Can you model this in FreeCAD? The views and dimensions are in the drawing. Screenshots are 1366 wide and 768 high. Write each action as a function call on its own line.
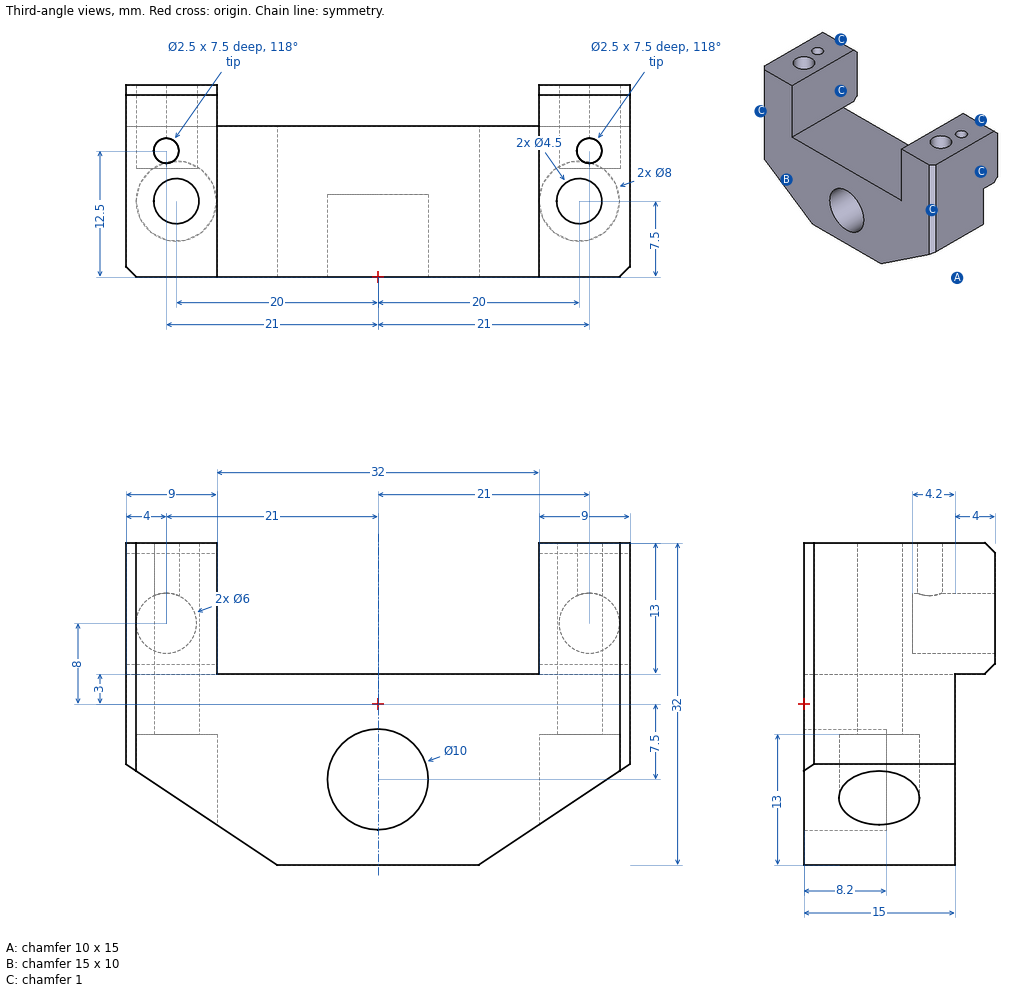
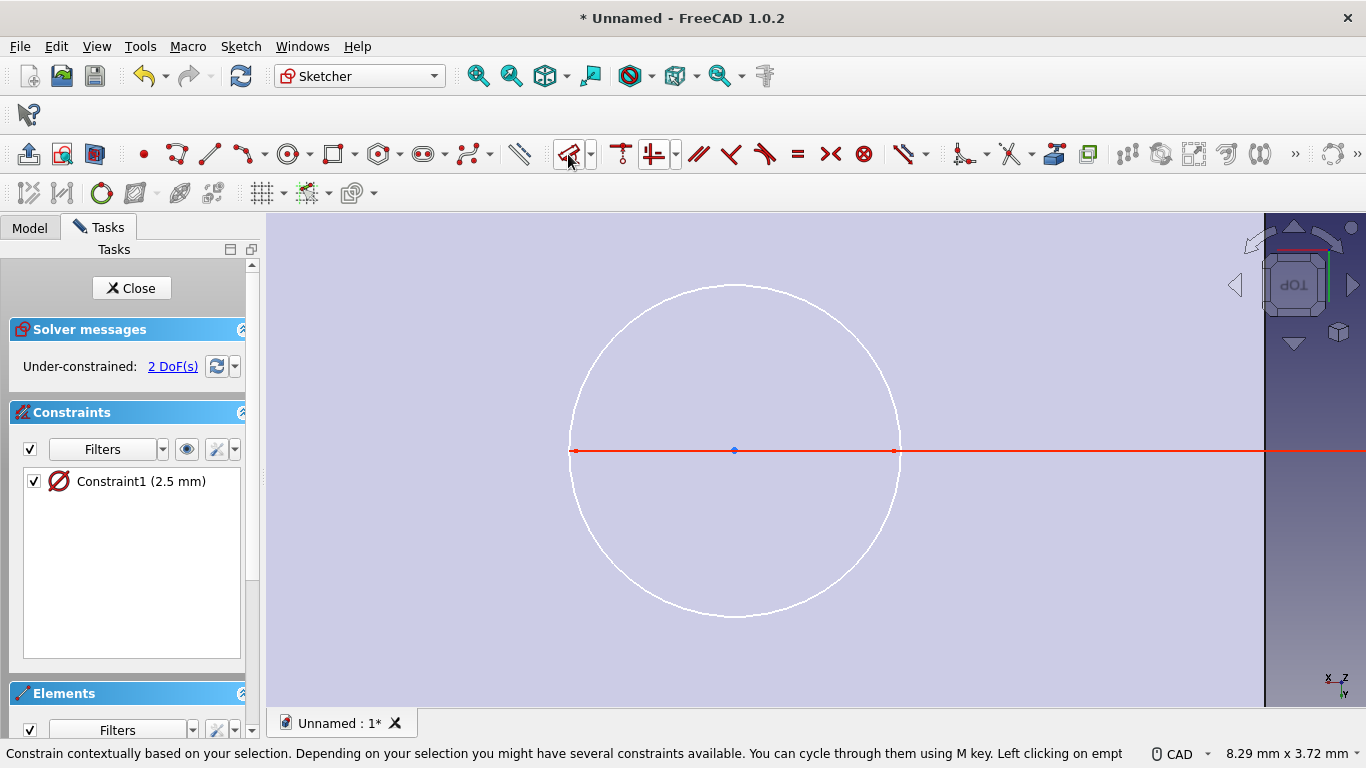
click(735, 451)
click(515, 485)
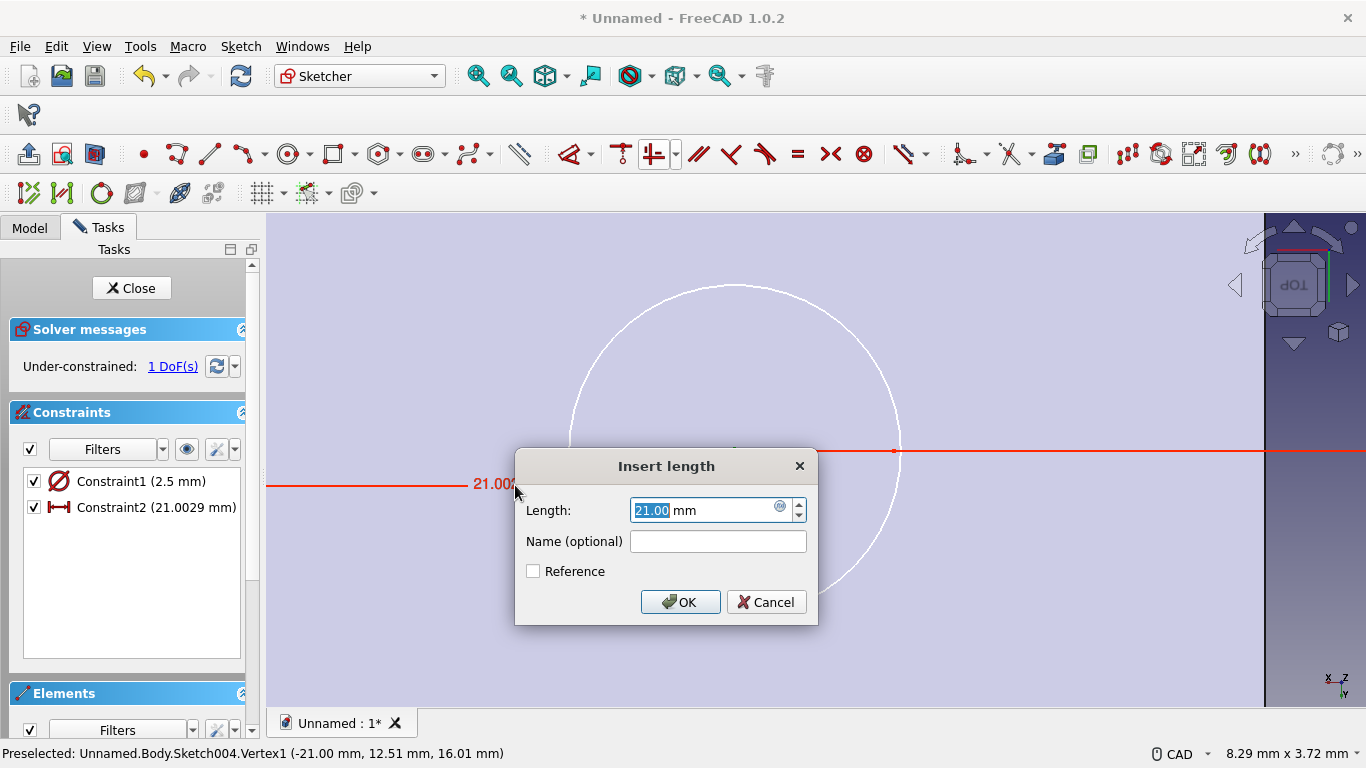
text(21)
key(Return)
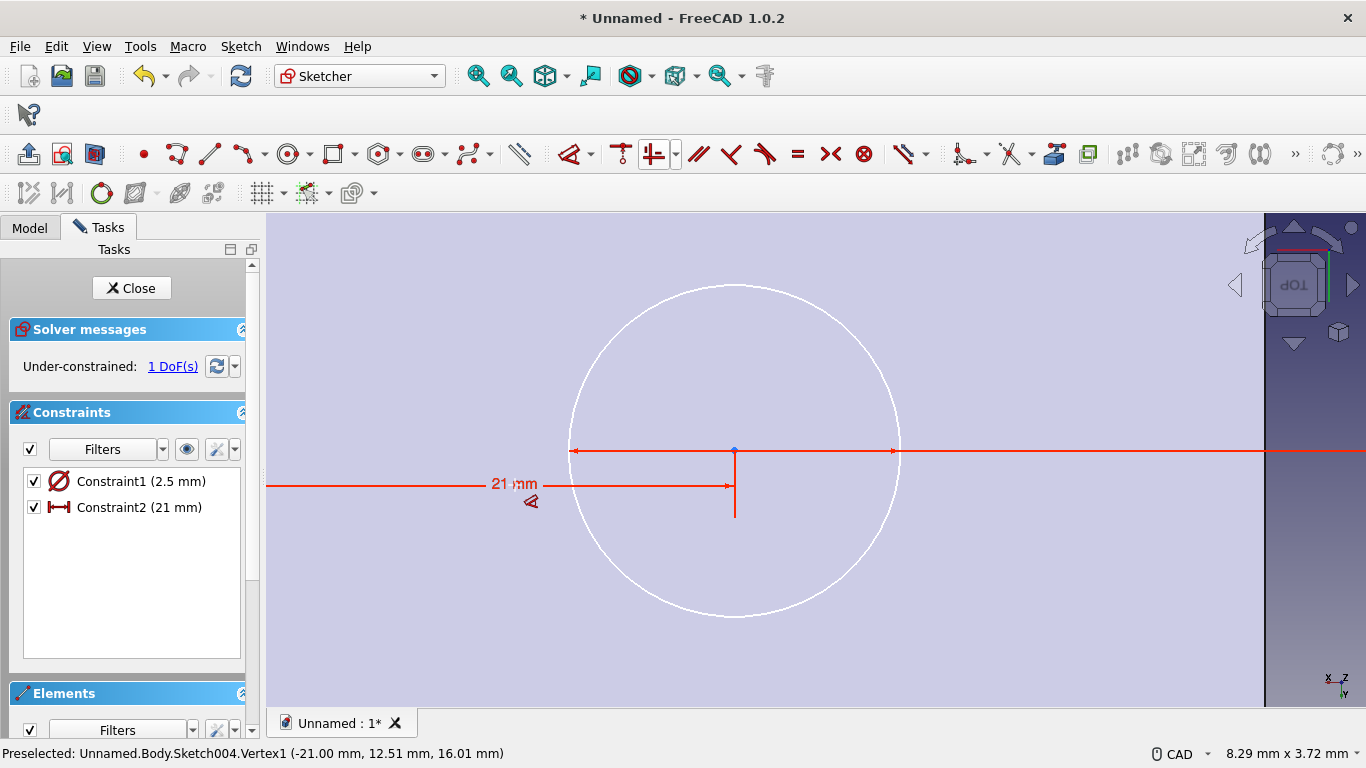
click(735, 451)
click(769, 346)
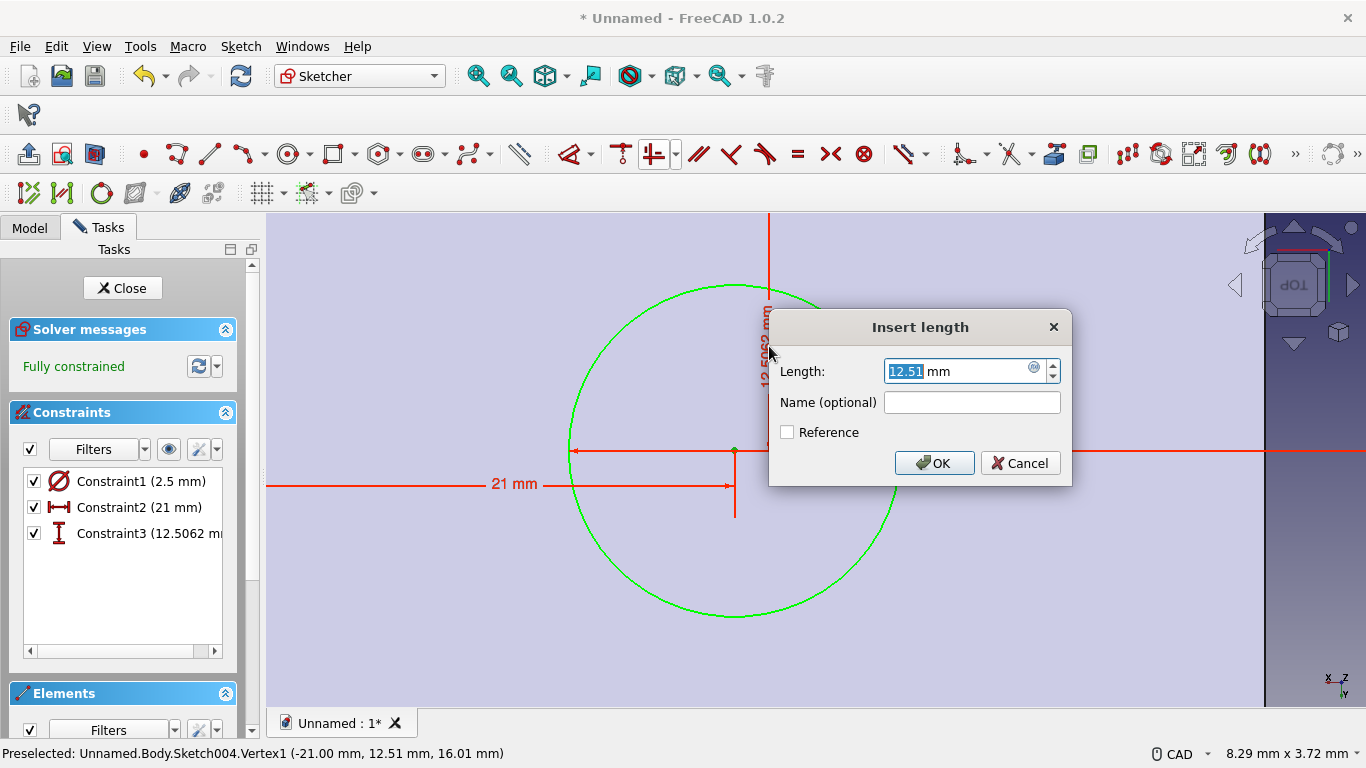
text(12.5)
key(Return)
key(Escape)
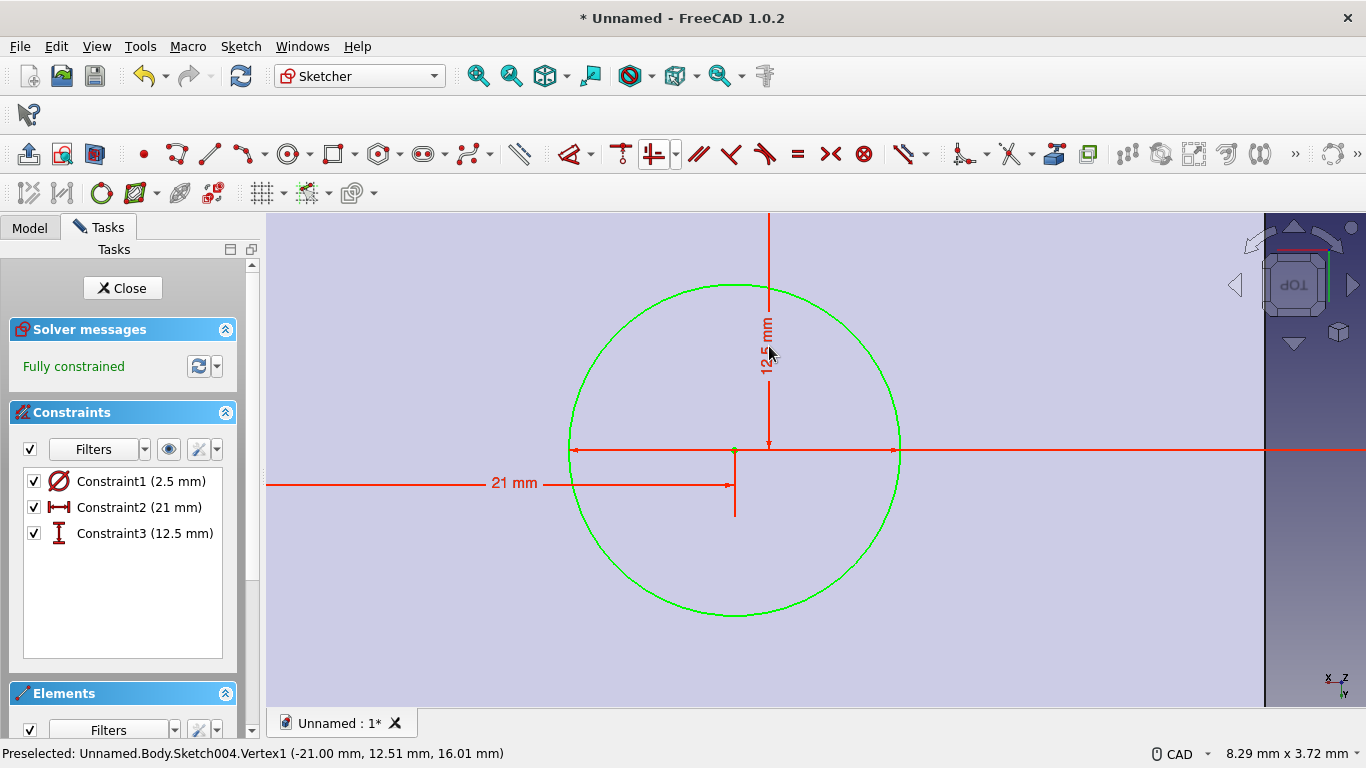
click(123, 288)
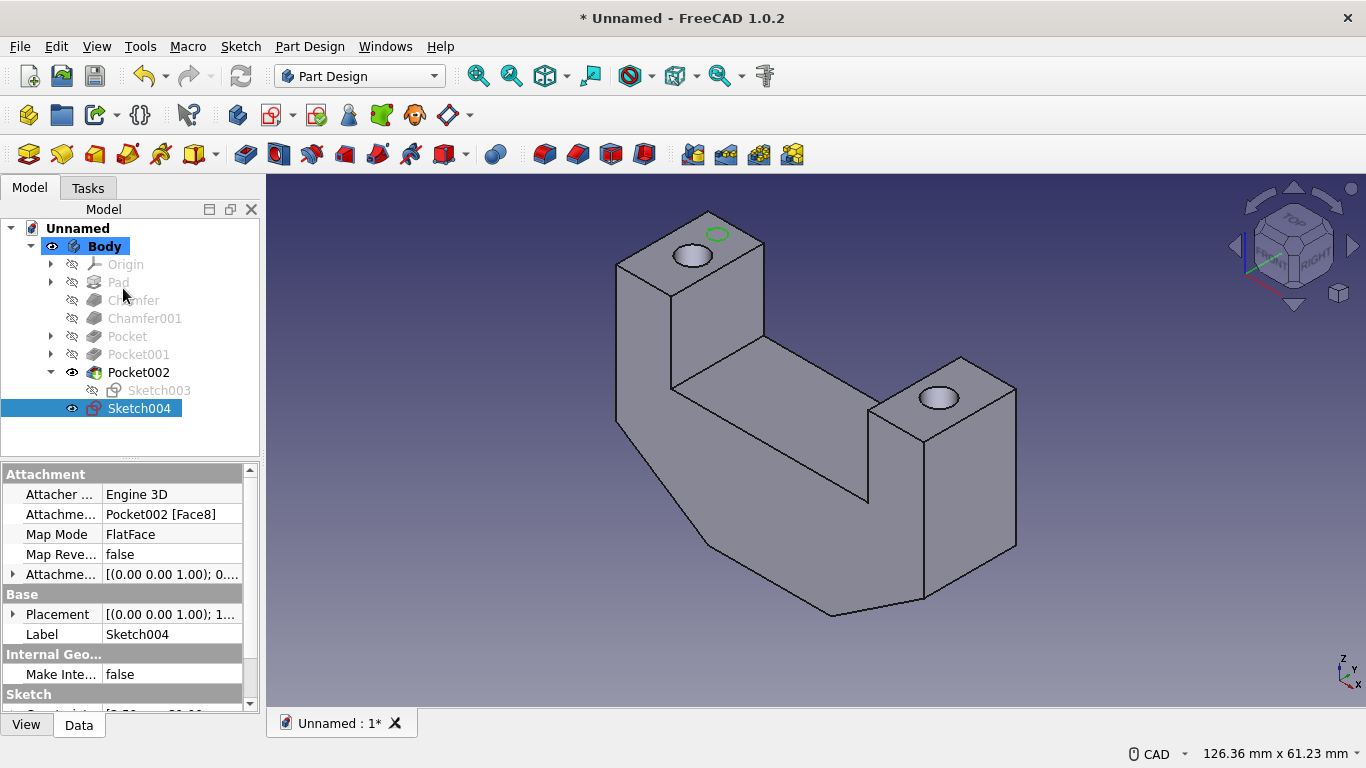
click(279, 154)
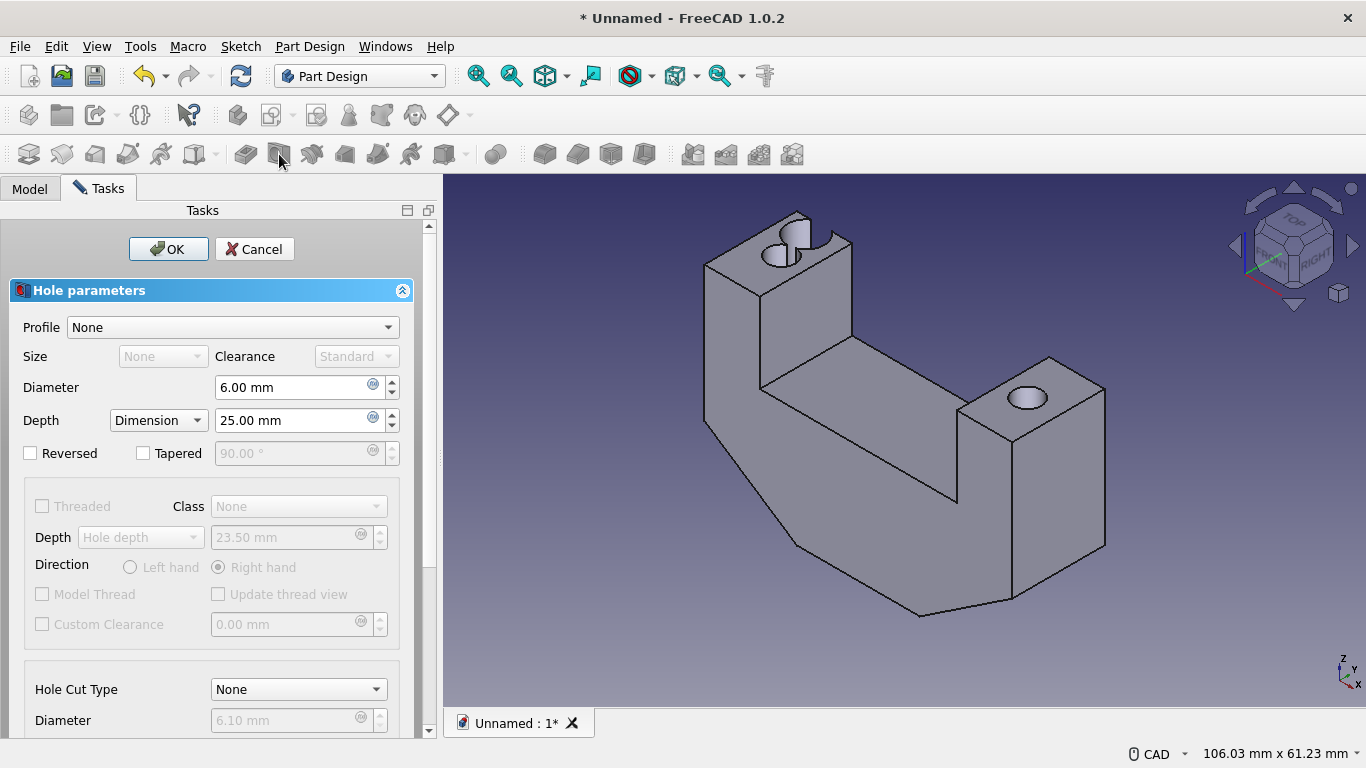
triple_click(300, 388)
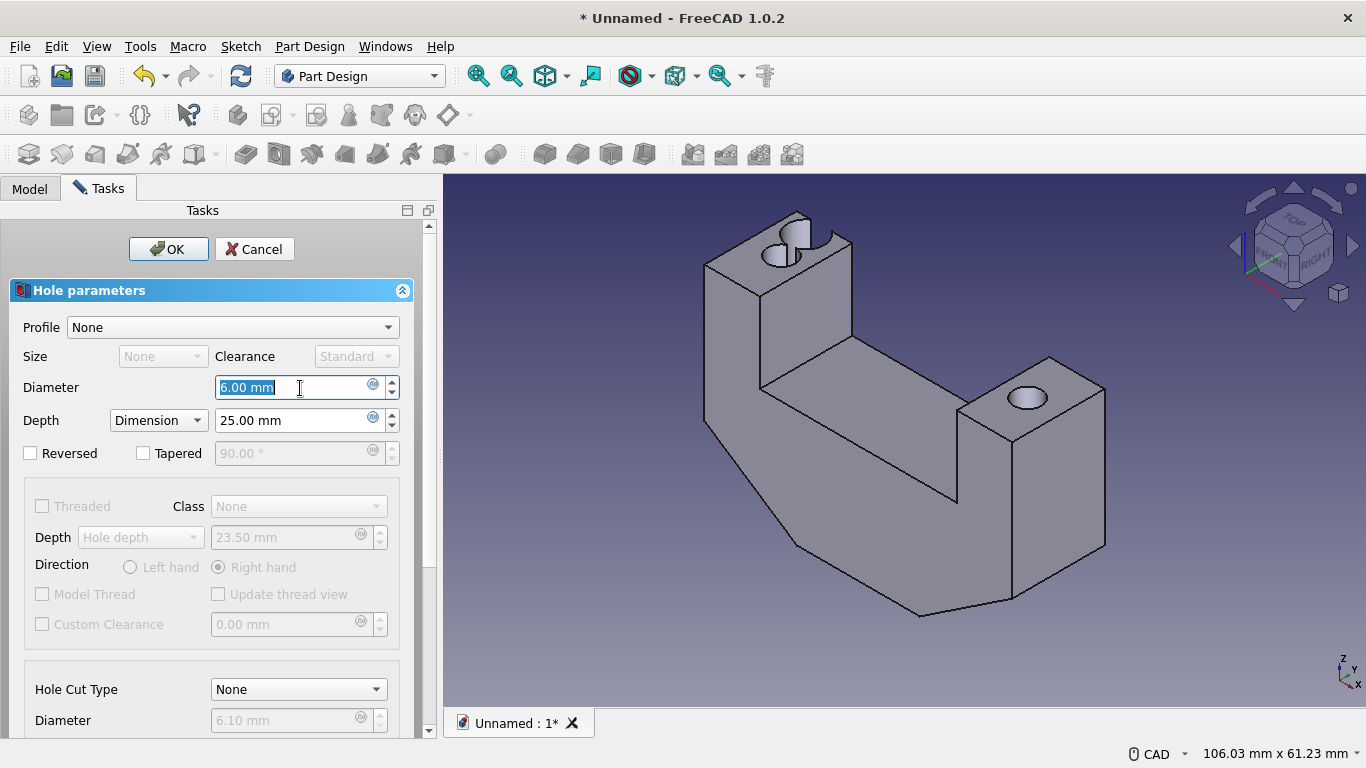
text(2.5)
key(Tab)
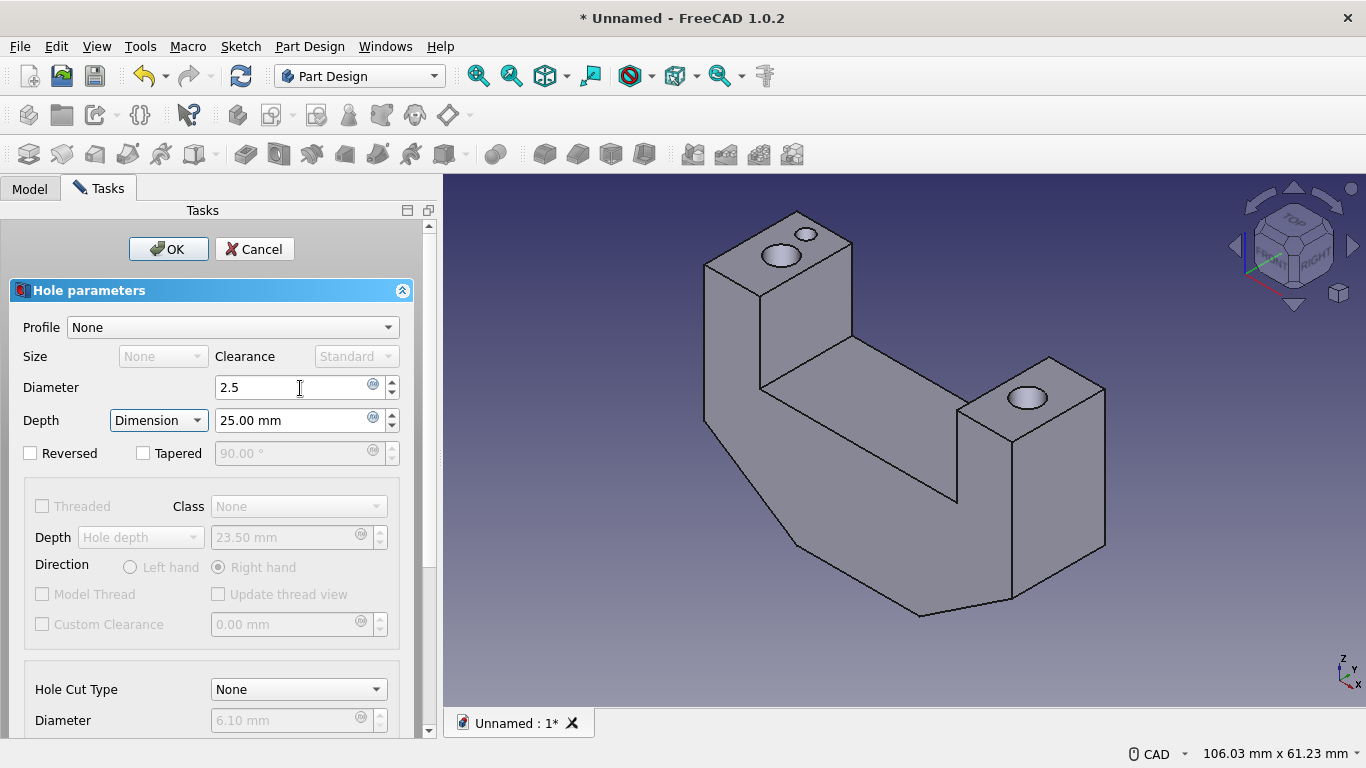
triple_click(300, 420)